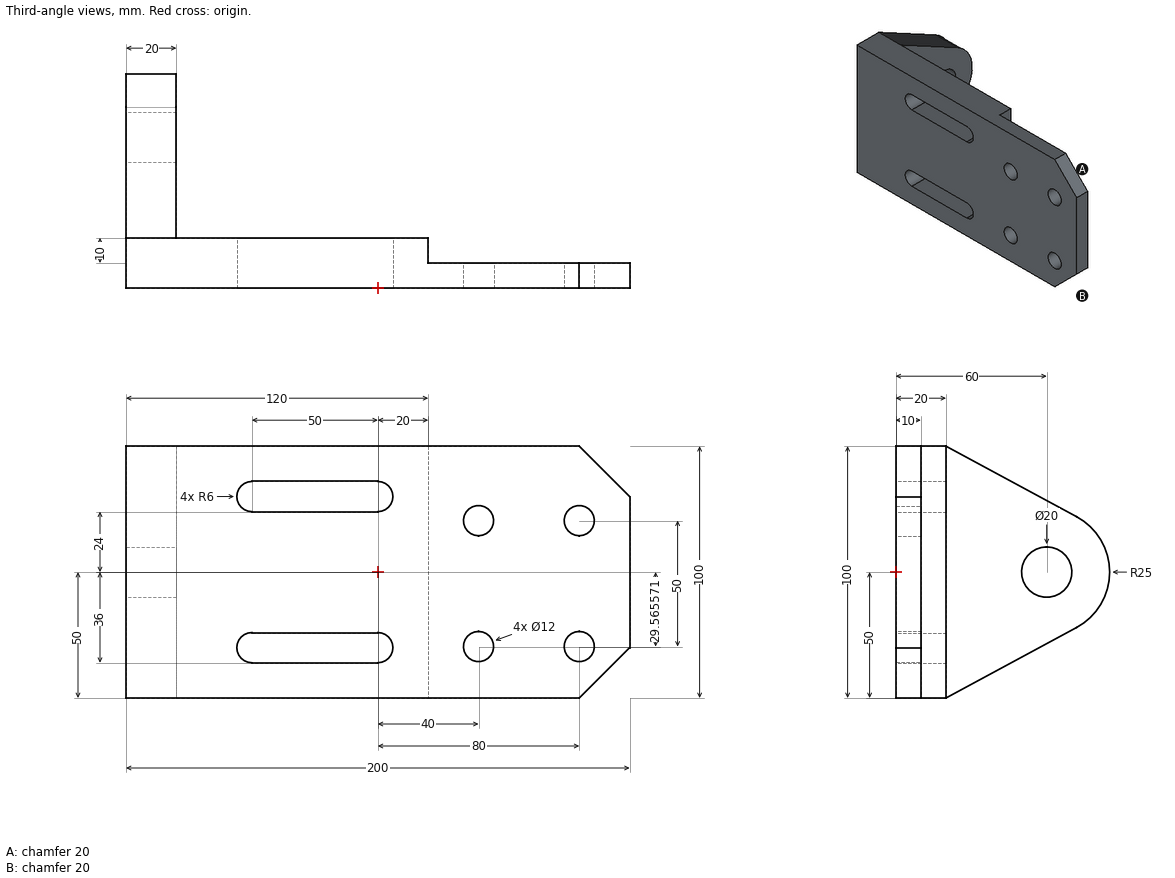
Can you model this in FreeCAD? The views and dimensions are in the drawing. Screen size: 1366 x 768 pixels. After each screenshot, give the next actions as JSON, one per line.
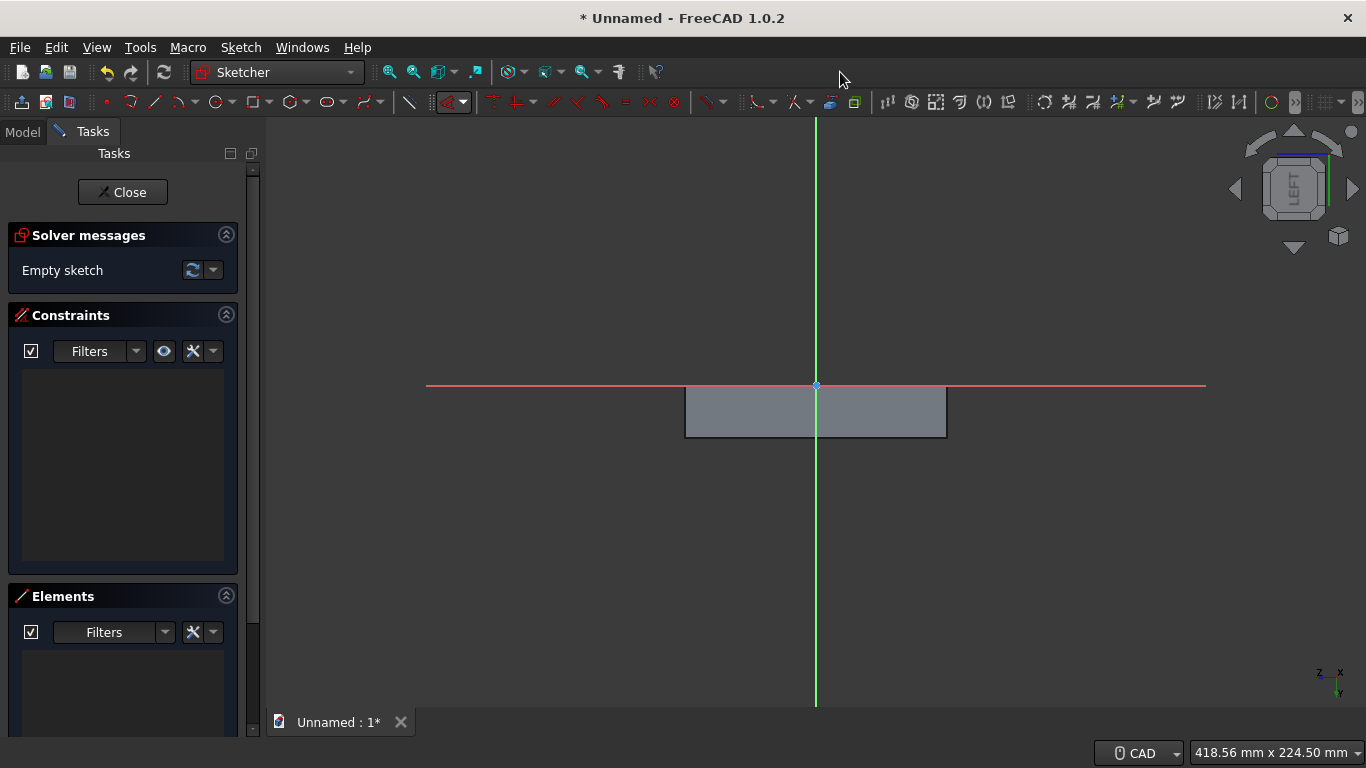
{"action": "scroll", "coordinate": [899, 601], "scroll_direction": "up", "scroll_amount": 3}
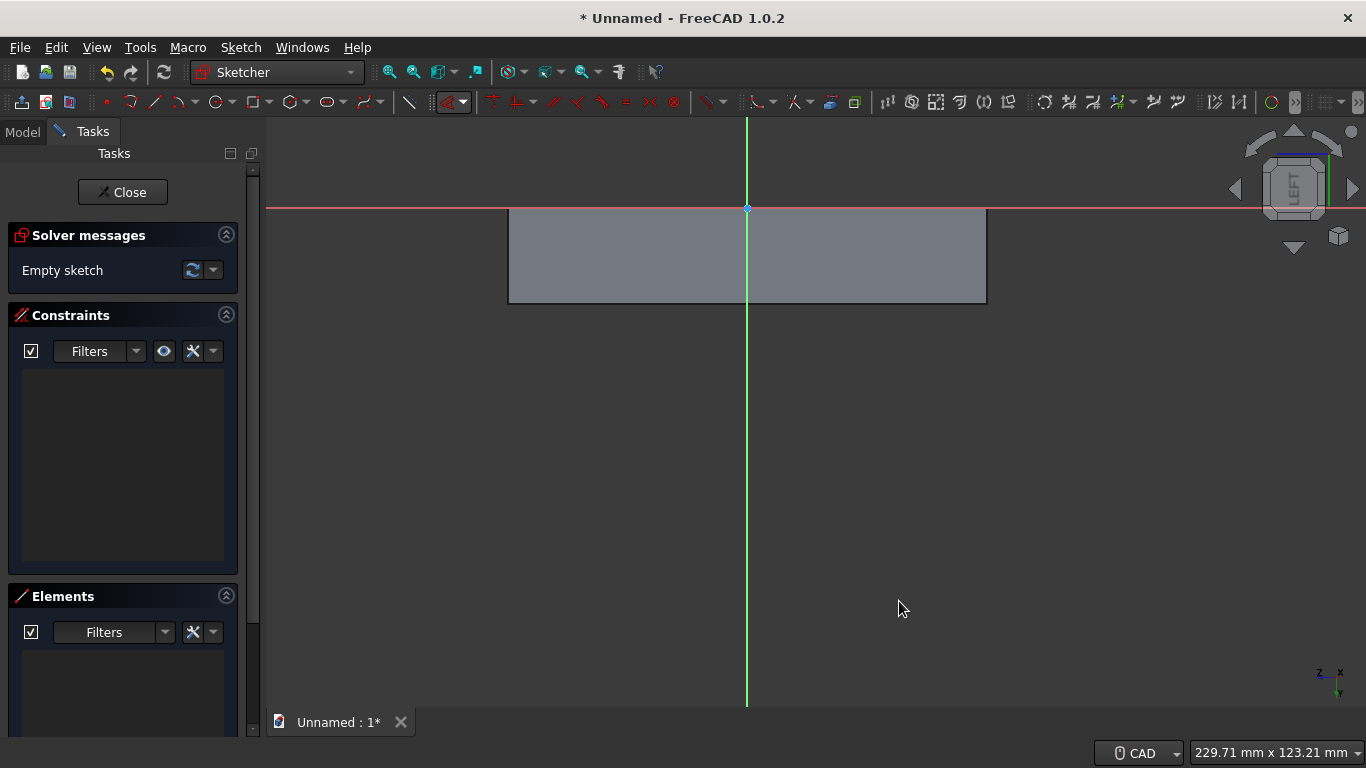
{"action": "left_click", "coordinate": [132, 102]}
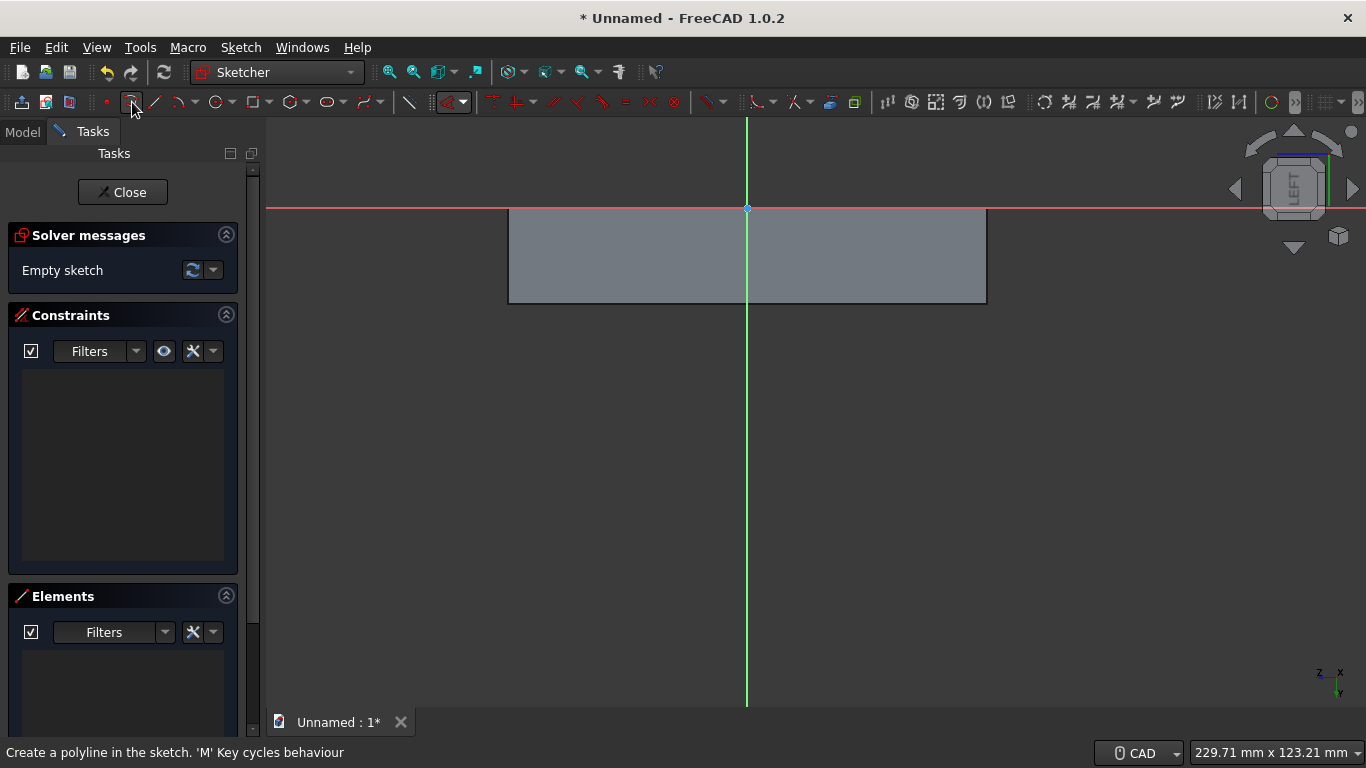
{"action": "left_click", "coordinate": [853, 552]}
{"action": "left_click", "coordinate": [987, 304]}
{"action": "left_click", "coordinate": [508, 304]}
{"action": "left_click", "coordinate": [642, 552]}
{"action": "right_click", "coordinate": [642, 552]}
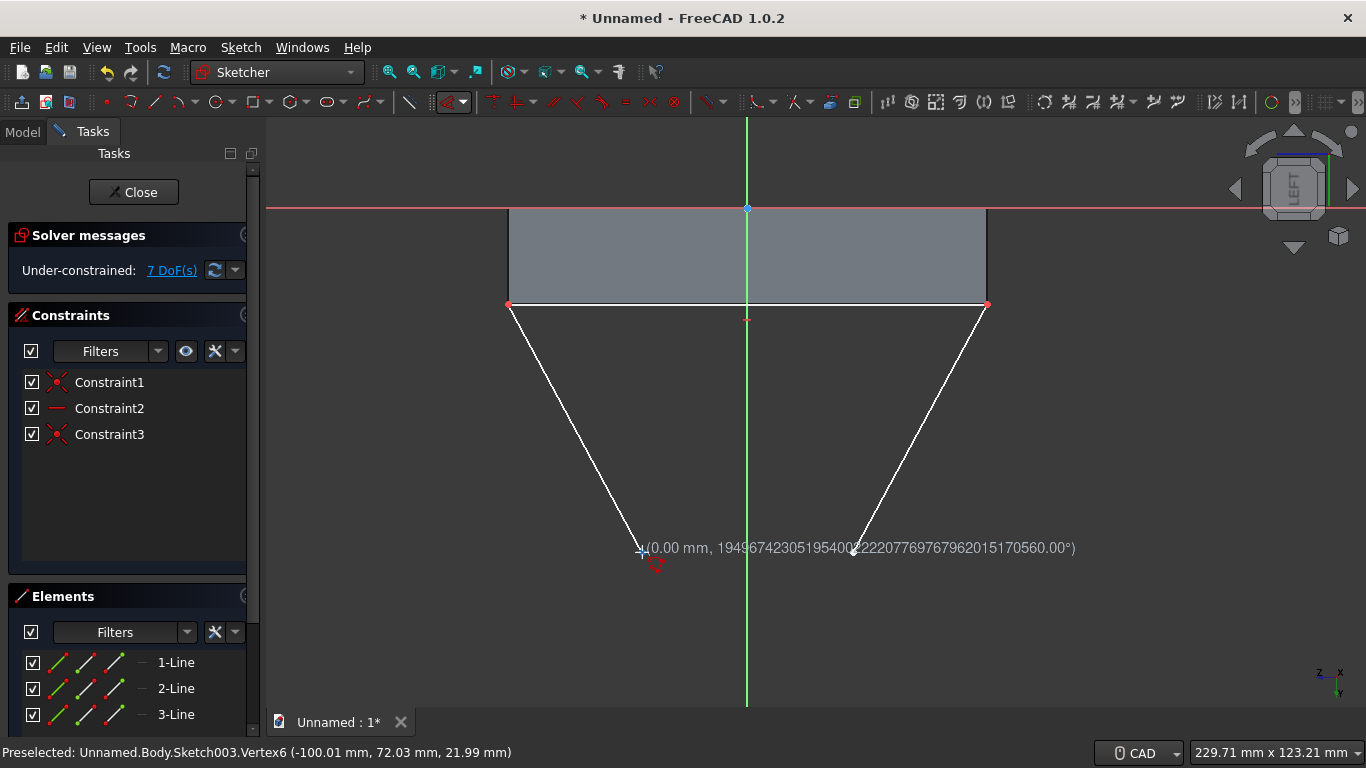
{"action": "key", "text": "g 3 a"}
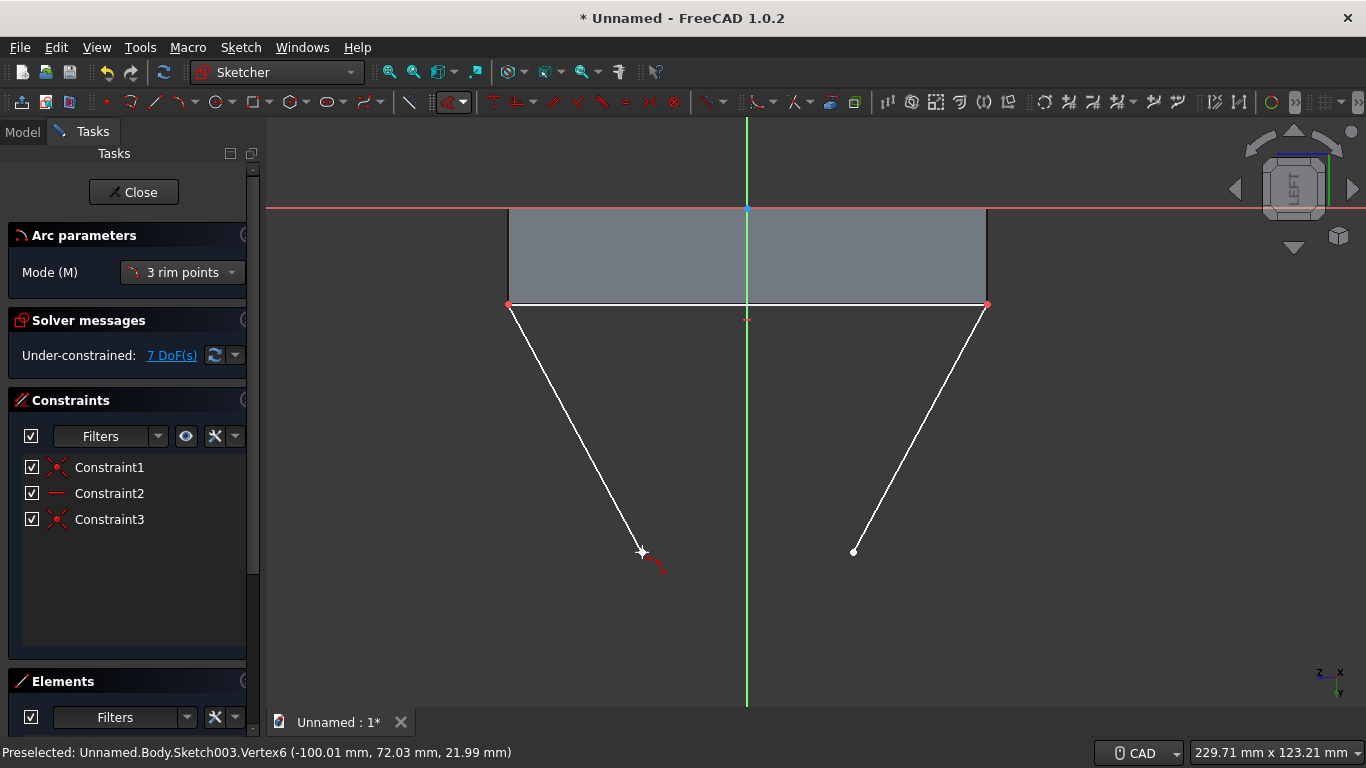
{"action": "left_click", "coordinate": [642, 553]}
{"action": "left_click", "coordinate": [853, 553]}
{"action": "left_click", "coordinate": [722, 612]}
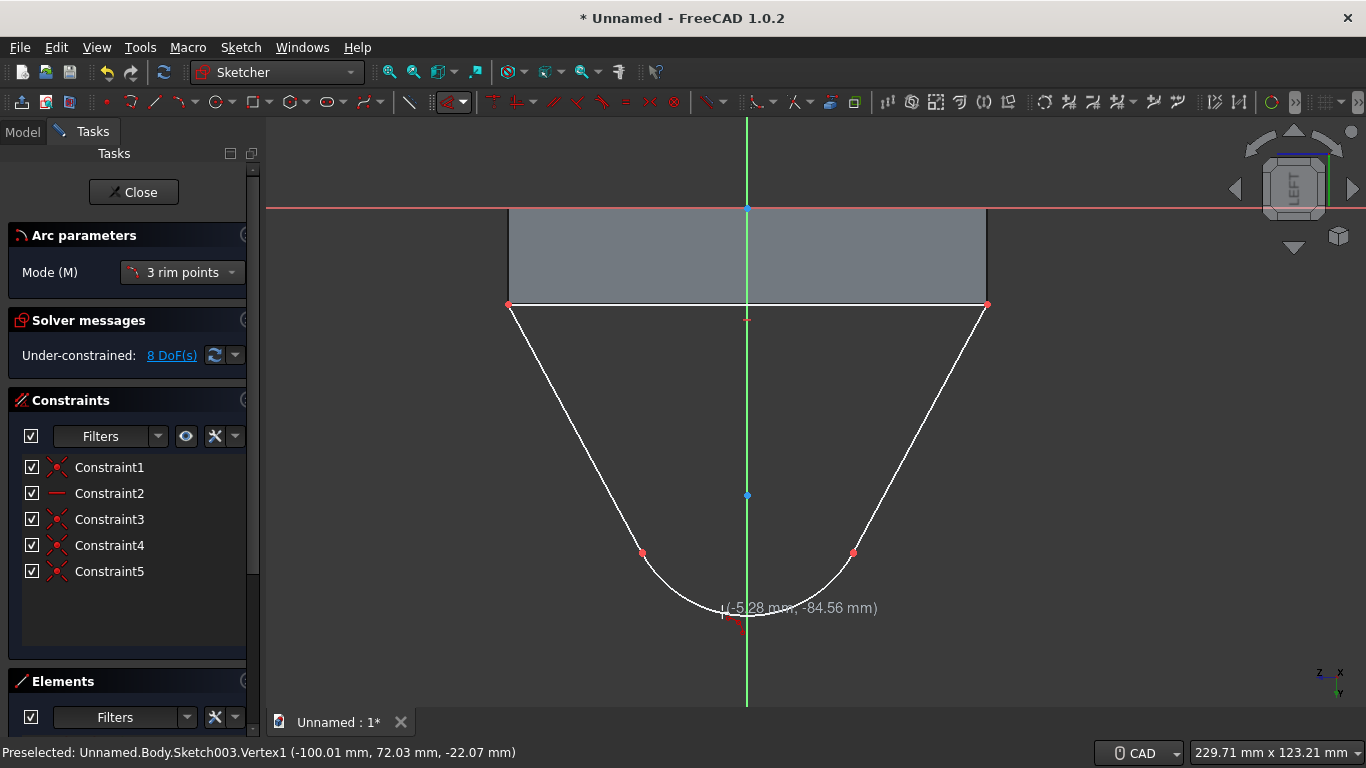
{"action": "left_click", "coordinate": [216, 102]}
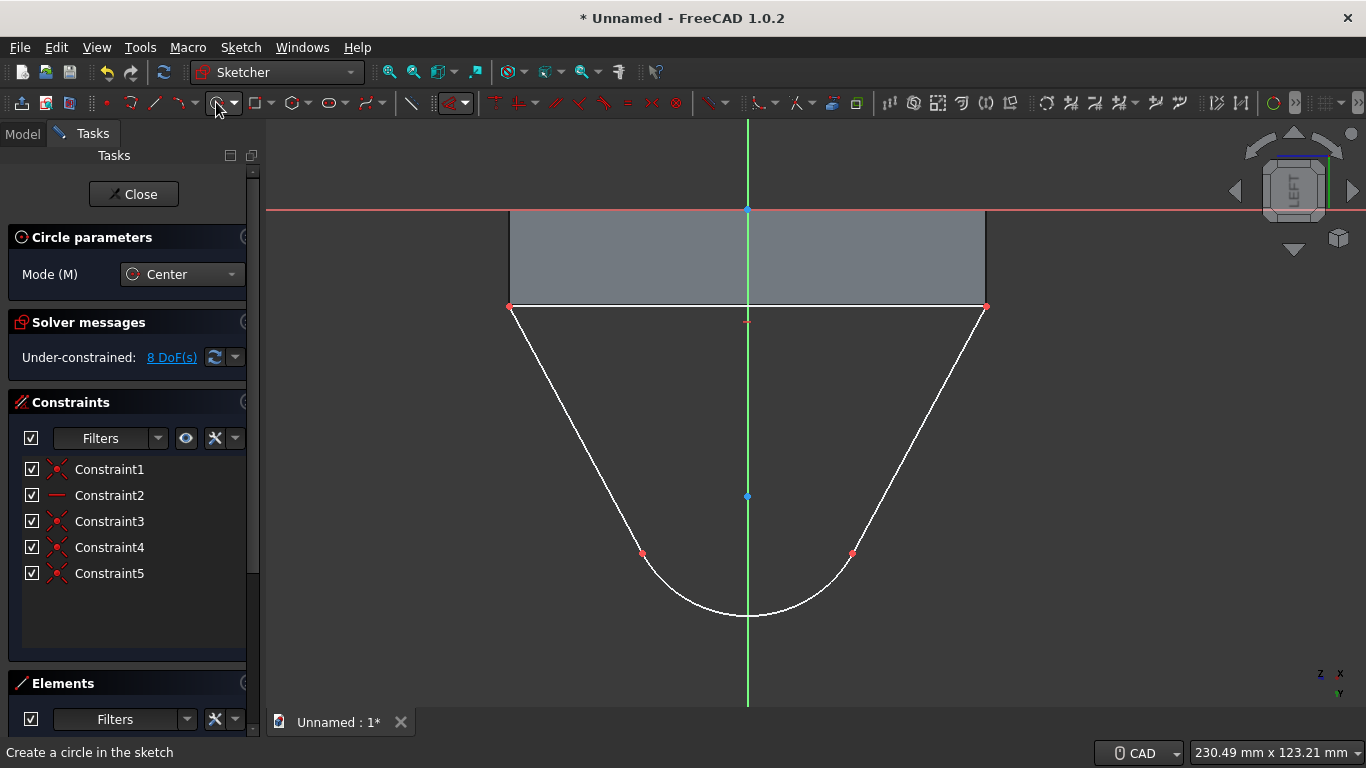
{"action": "left_click", "coordinate": [748, 496]}
{"action": "mouse_move", "coordinate": [781, 462]}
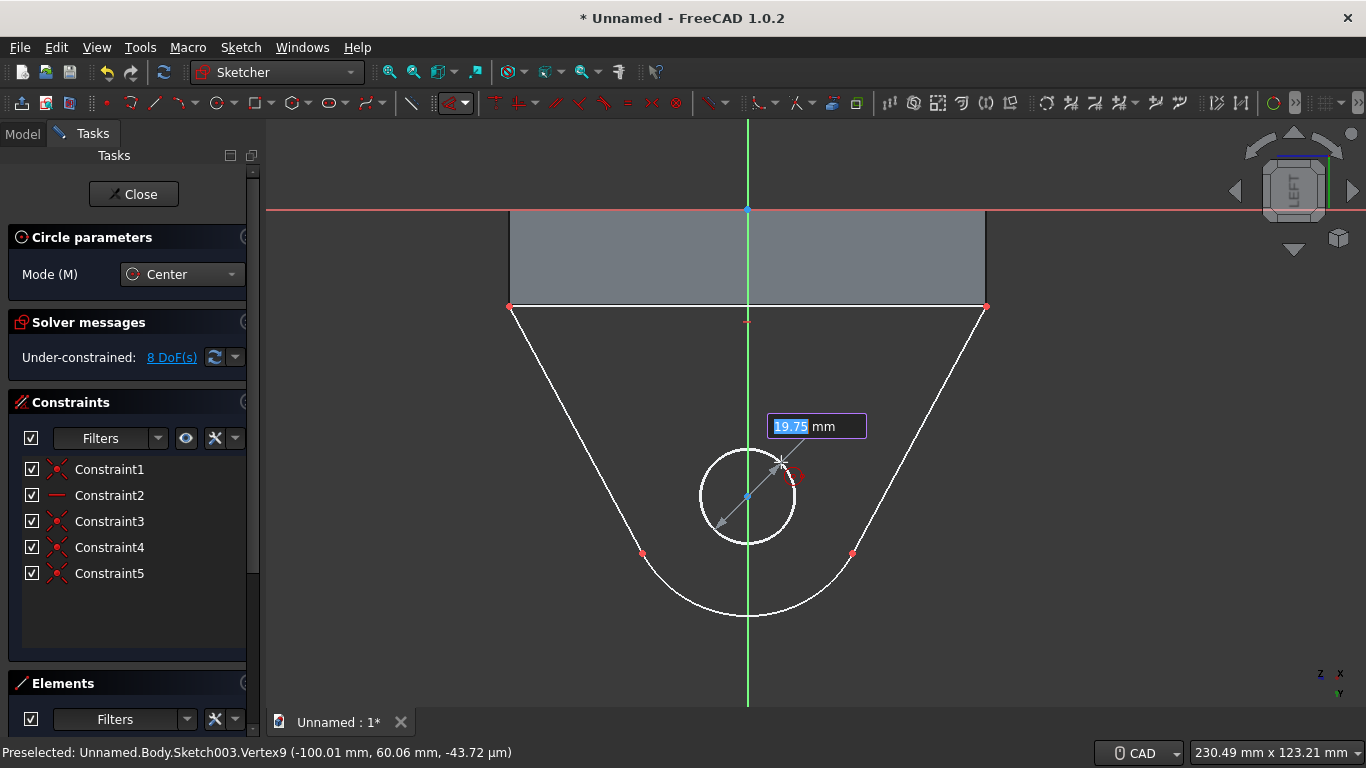
{"action": "type", "text": "20"}
{"action": "key", "text": "Return"}
{"action": "key", "text": "Escape"}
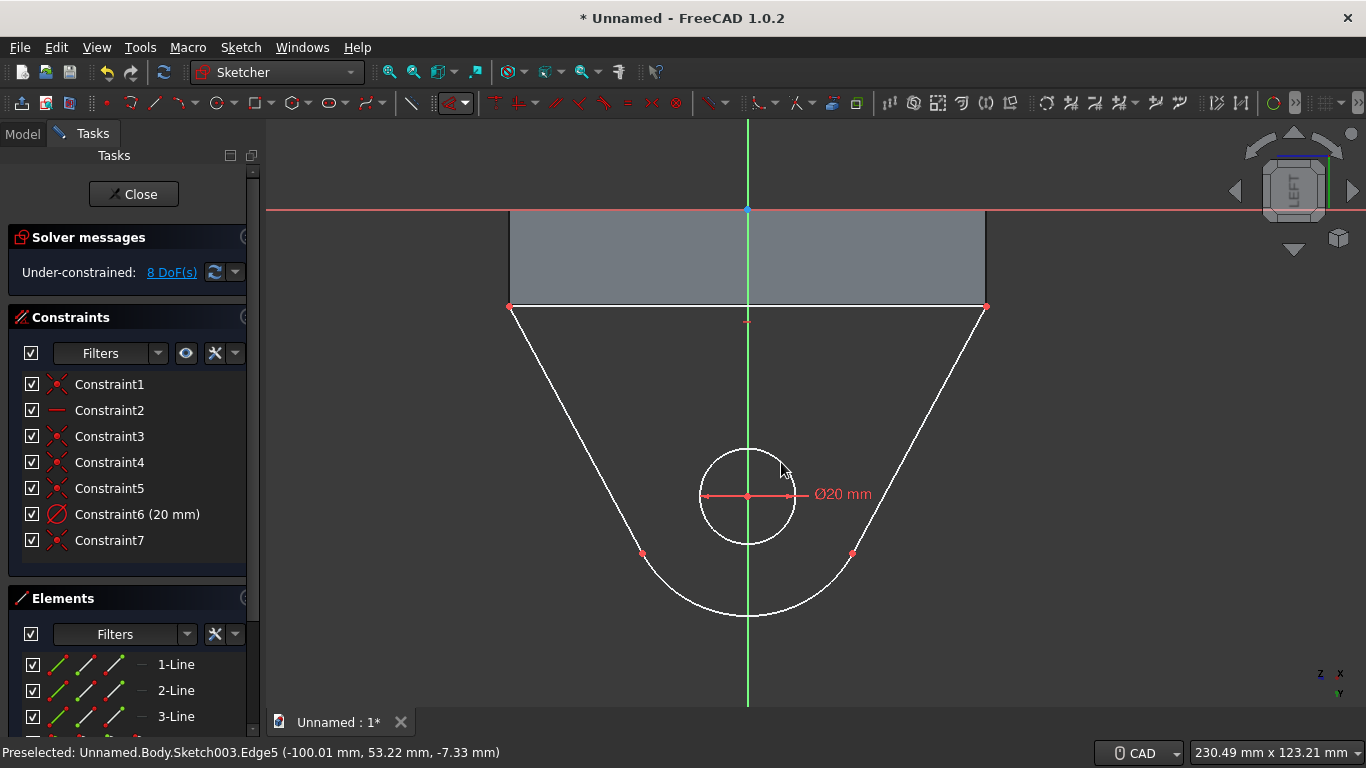
{"action": "left_click", "coordinate": [893, 479]}